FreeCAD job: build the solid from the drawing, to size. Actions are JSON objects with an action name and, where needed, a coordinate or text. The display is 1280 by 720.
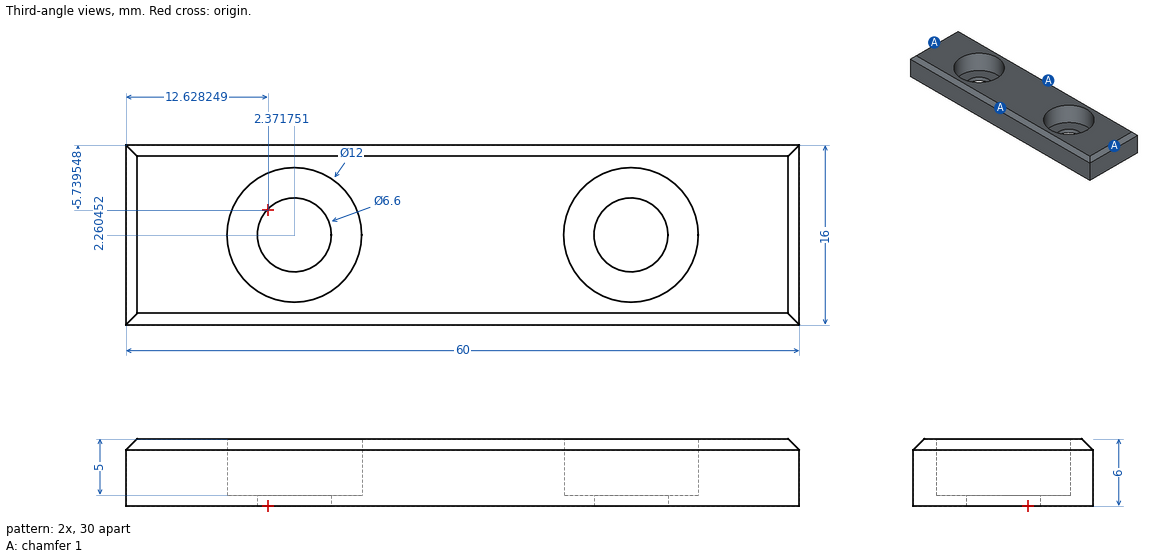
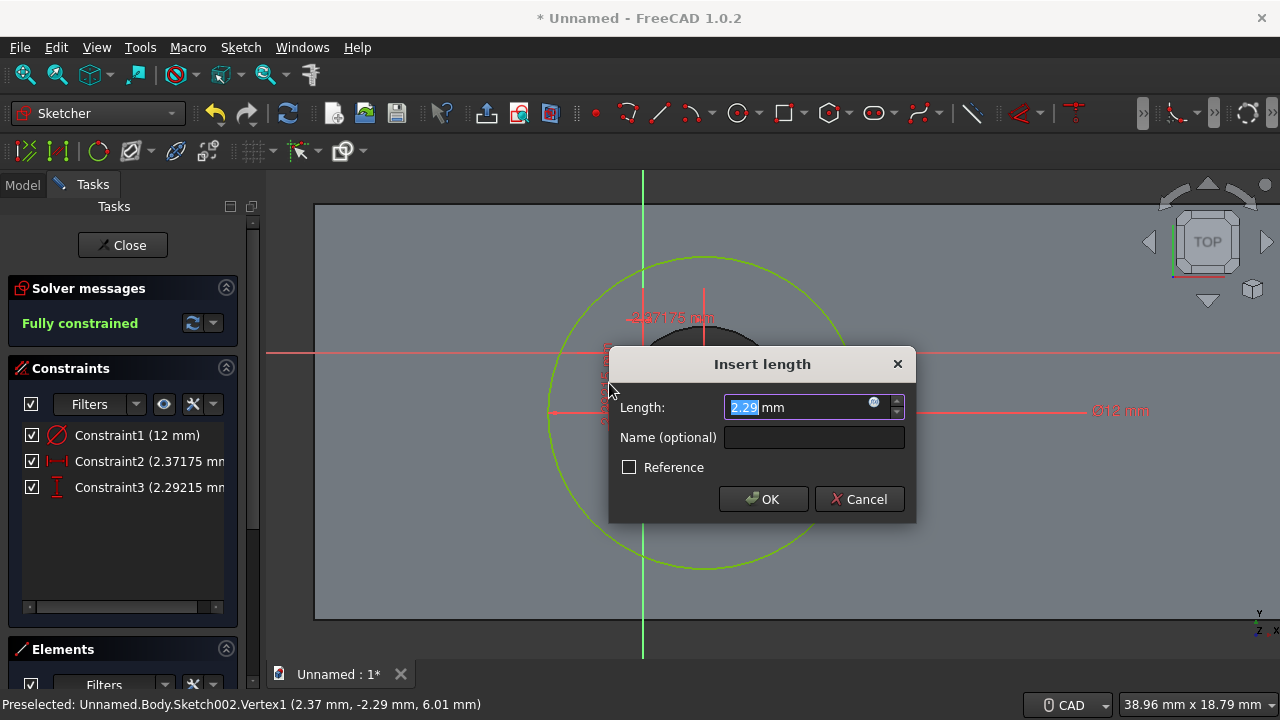
{"action": "type", "text": "2.260452"}
{"action": "key", "text": "Return"}
{"action": "key", "text": "Escape"}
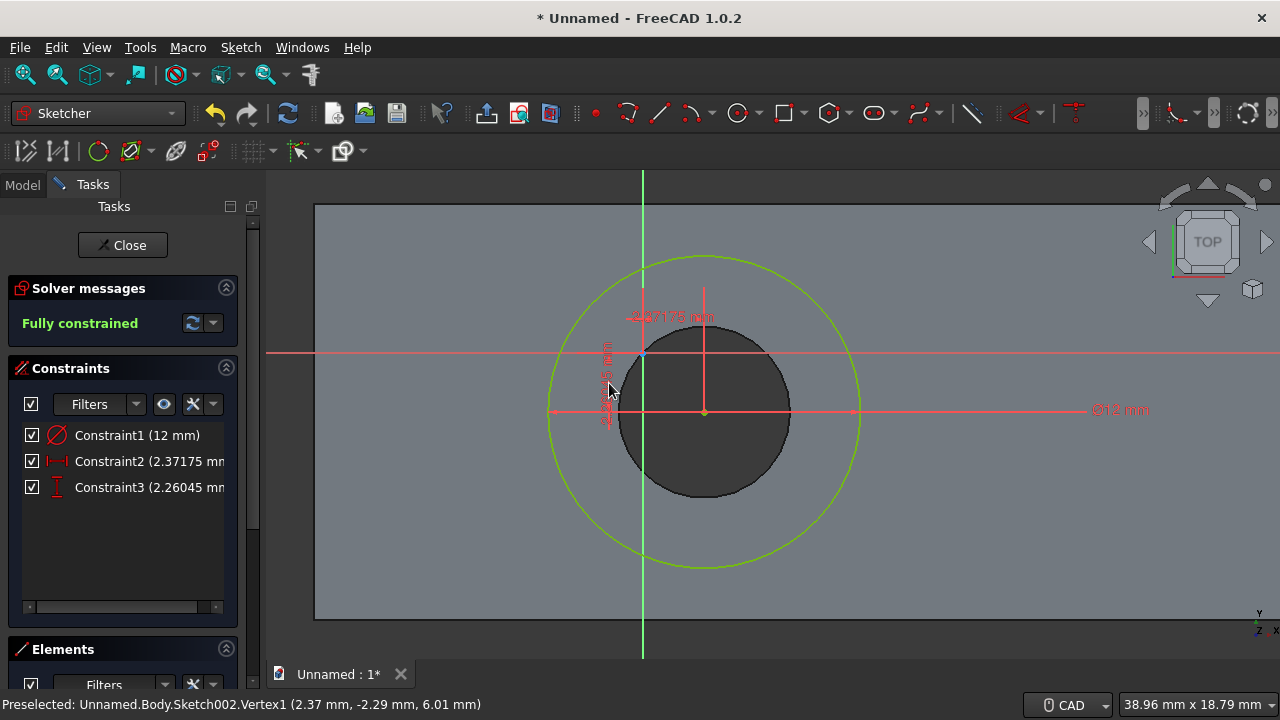
{"action": "left_click", "coordinate": [123, 245]}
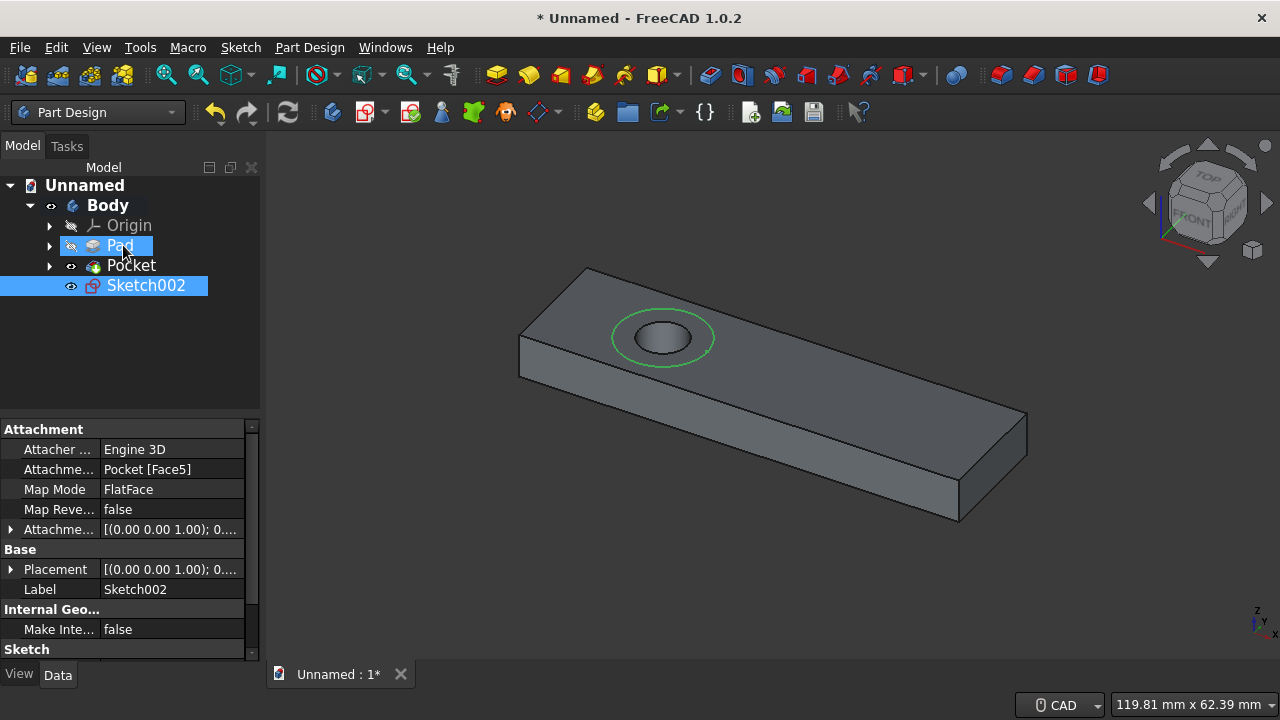
{"action": "left_click", "coordinate": [712, 76]}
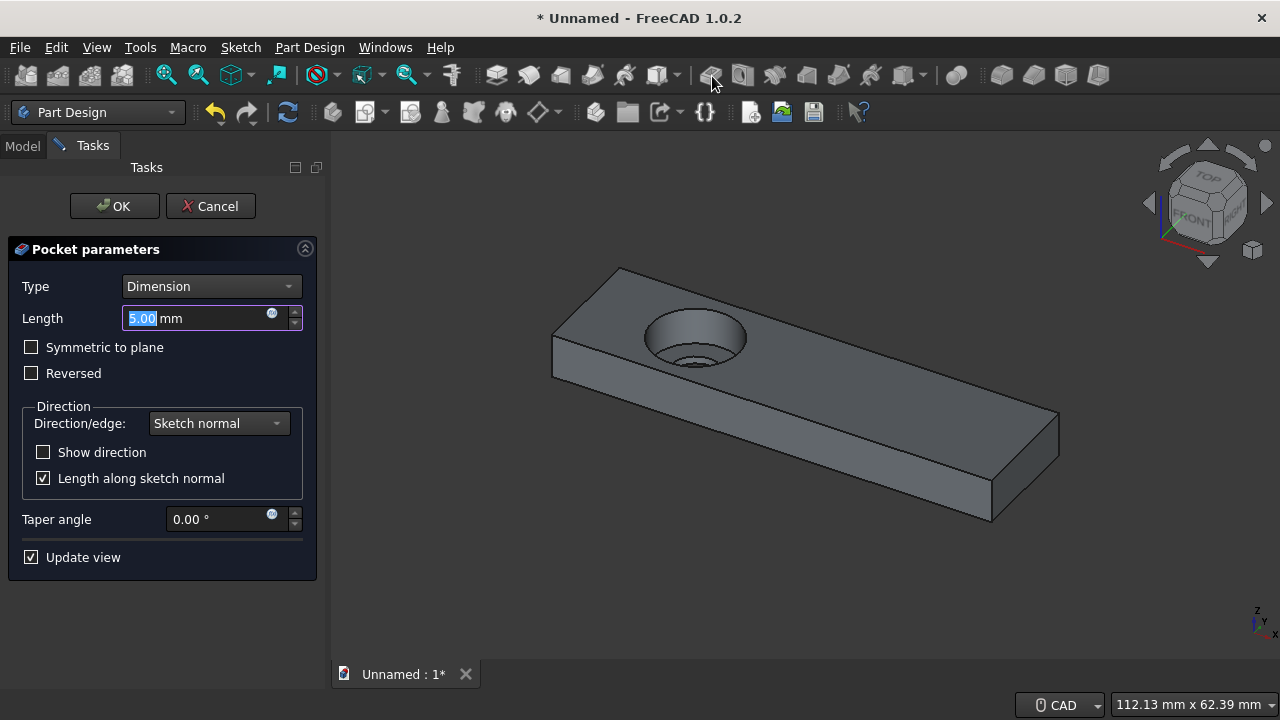
{"action": "type", "text": "5"}
{"action": "key", "text": "Tab"}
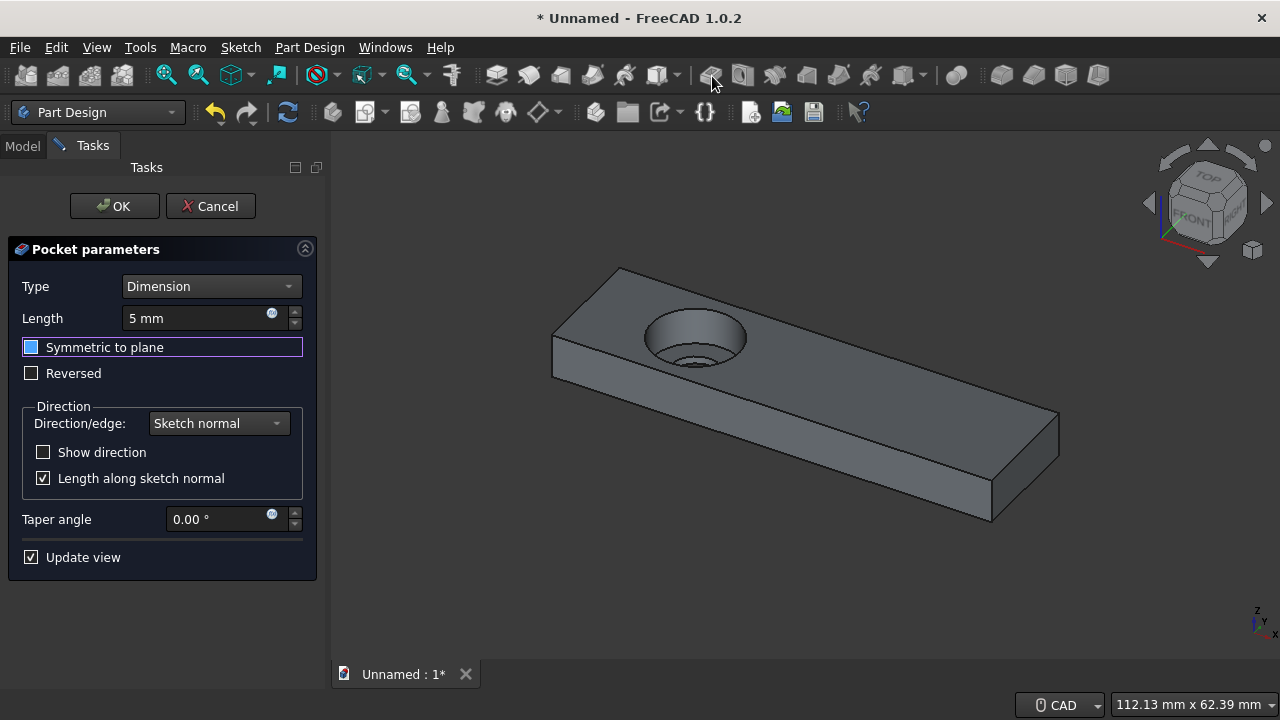
{"action": "left_click", "coordinate": [115, 206]}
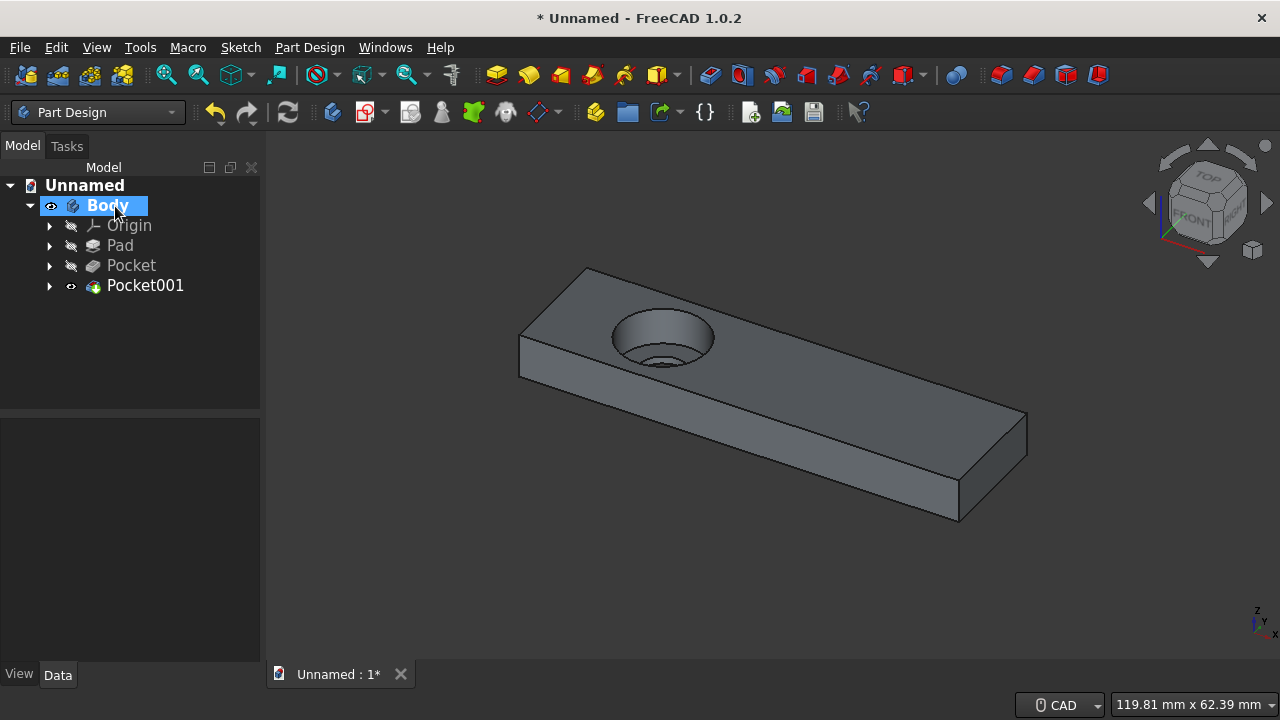
{"action": "left_click", "coordinate": [116, 266]}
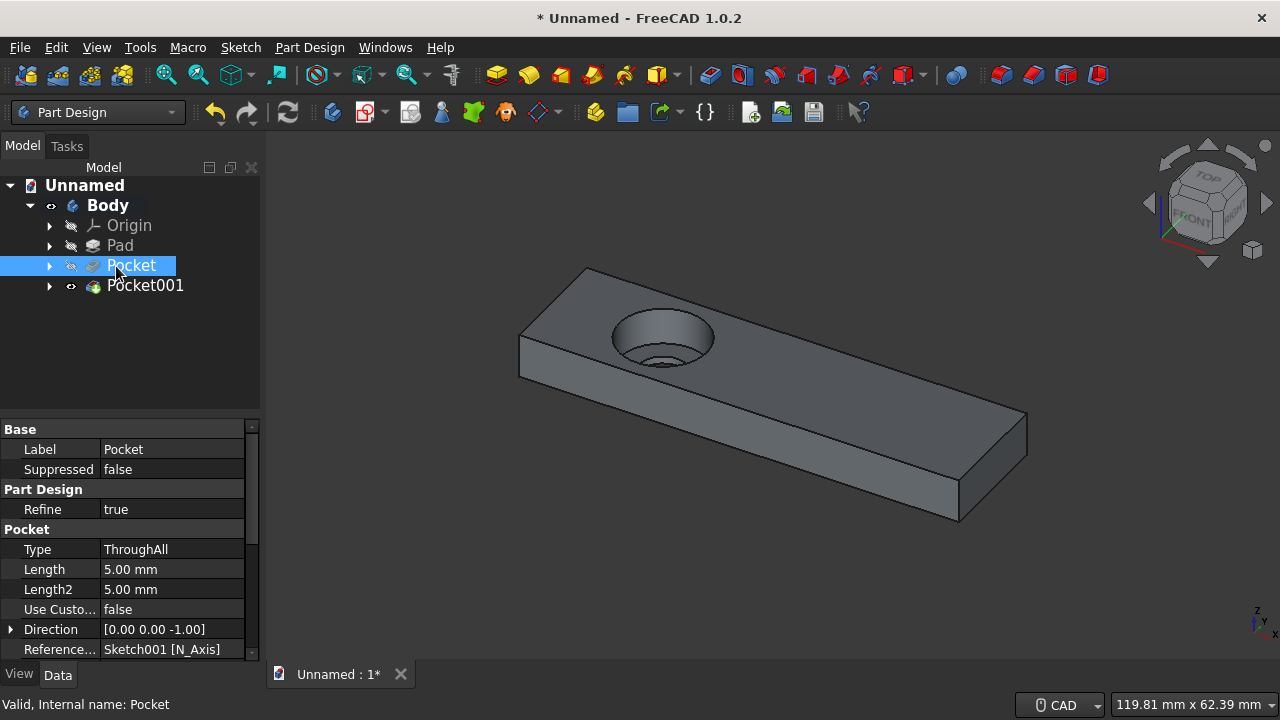
{"action": "left_click", "coordinate": [116, 286], "text": "ctrl"}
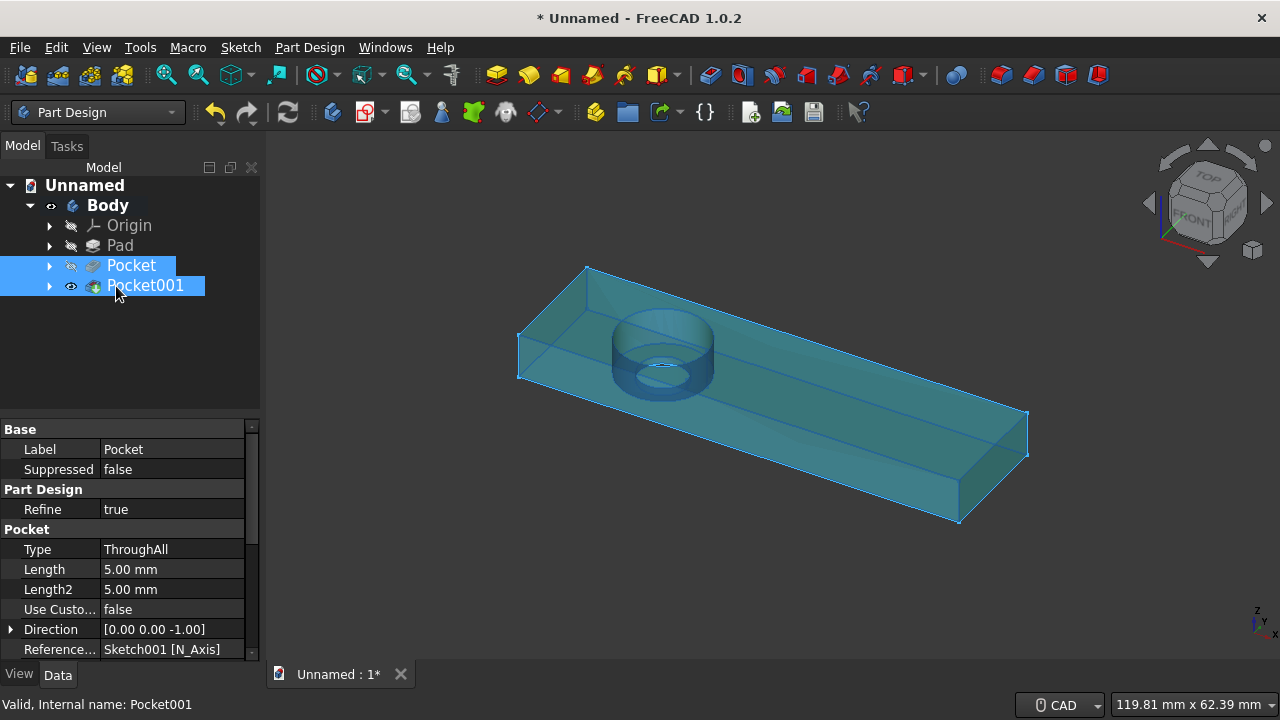
{"action": "left_click", "coordinate": [58, 76]}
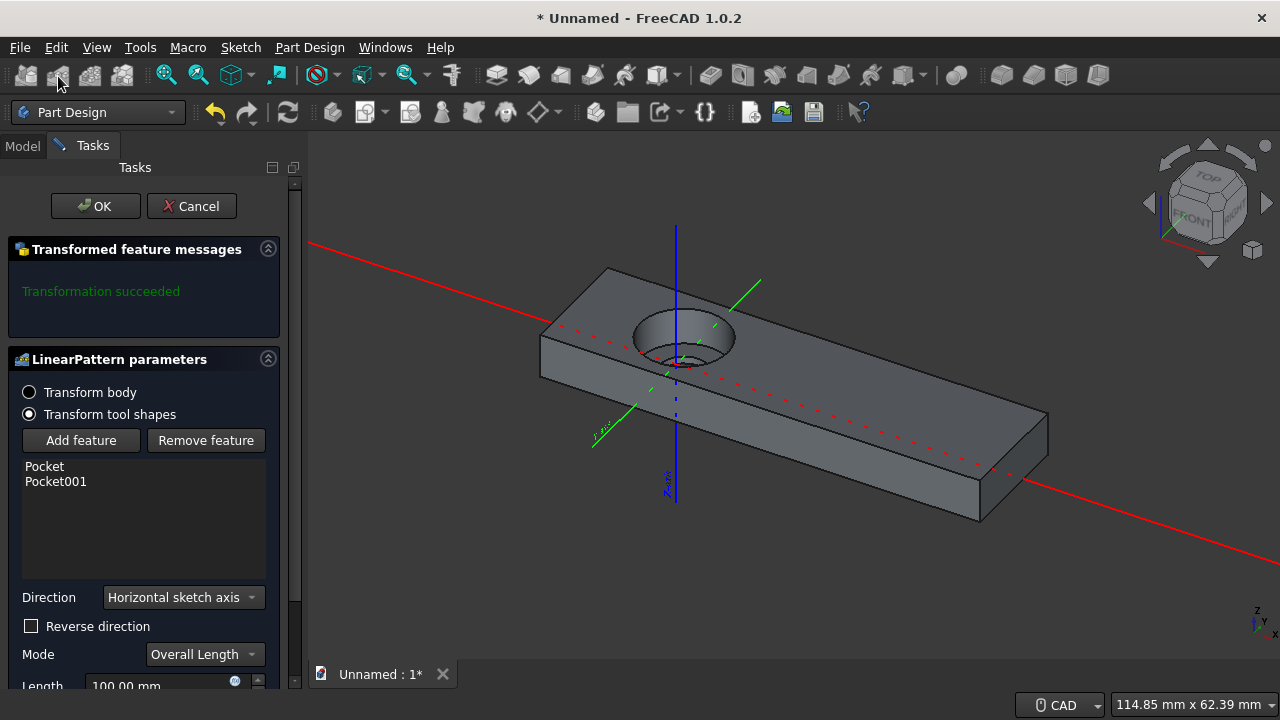
{"action": "left_click", "coordinate": [184, 598]}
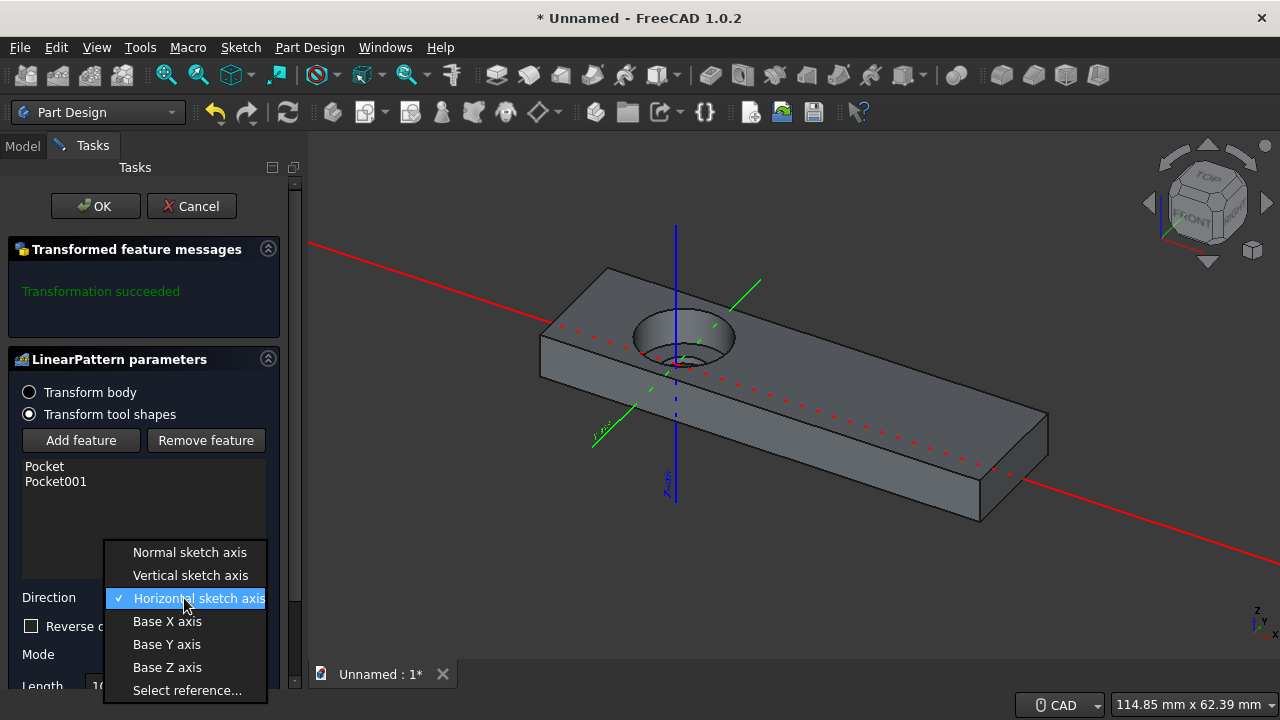
{"action": "left_click", "coordinate": [184, 622]}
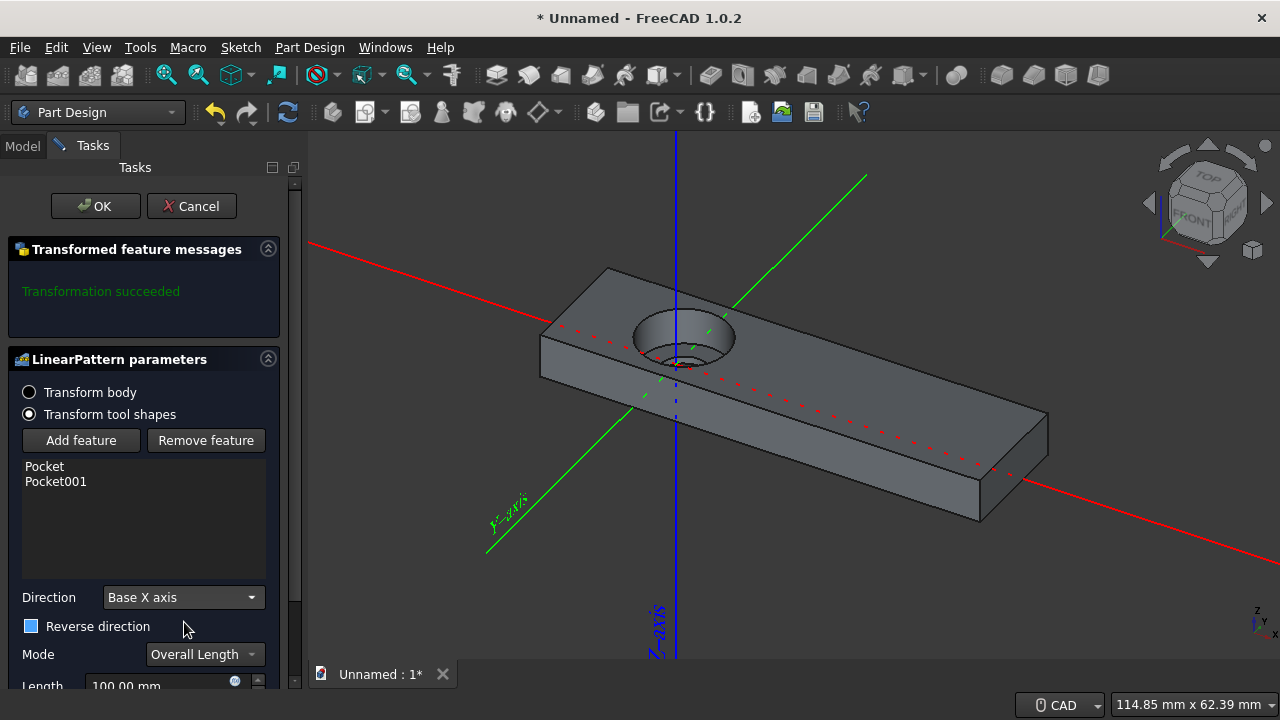
{"action": "left_click", "coordinate": [206, 654]}